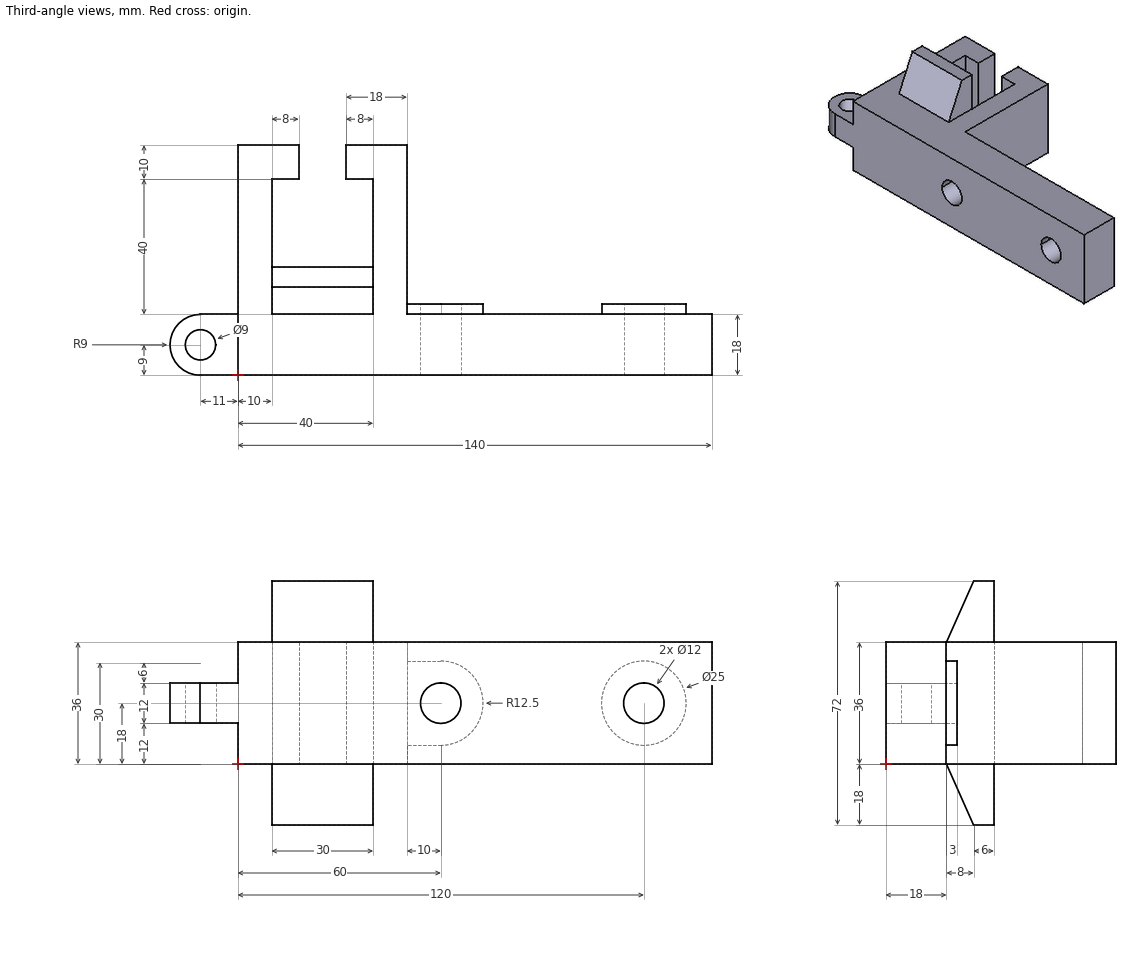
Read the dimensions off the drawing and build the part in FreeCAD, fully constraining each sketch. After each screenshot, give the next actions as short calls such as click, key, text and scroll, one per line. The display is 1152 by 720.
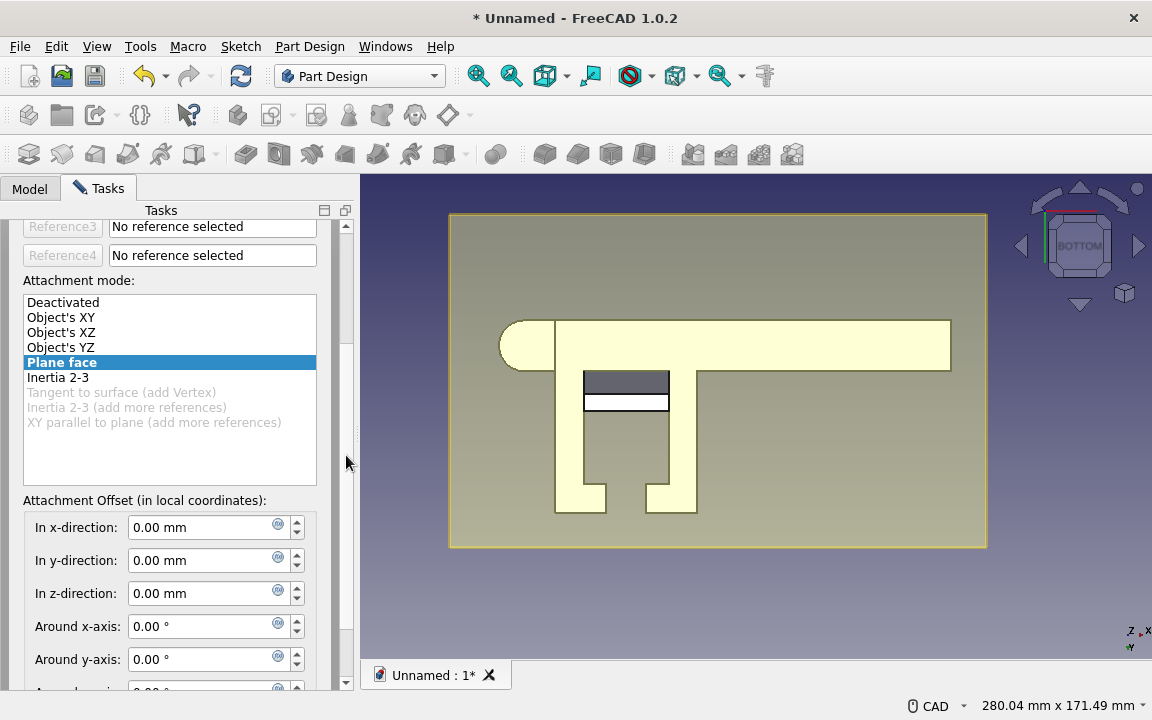
triple_click(210, 594)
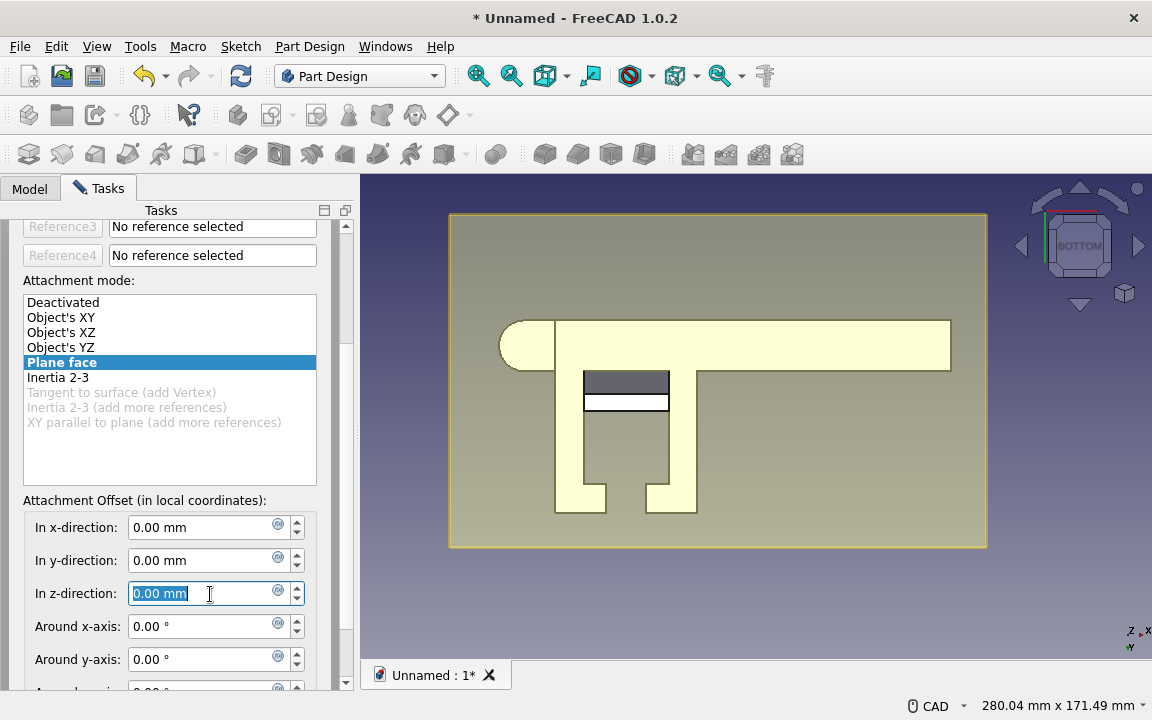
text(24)
key(Tab)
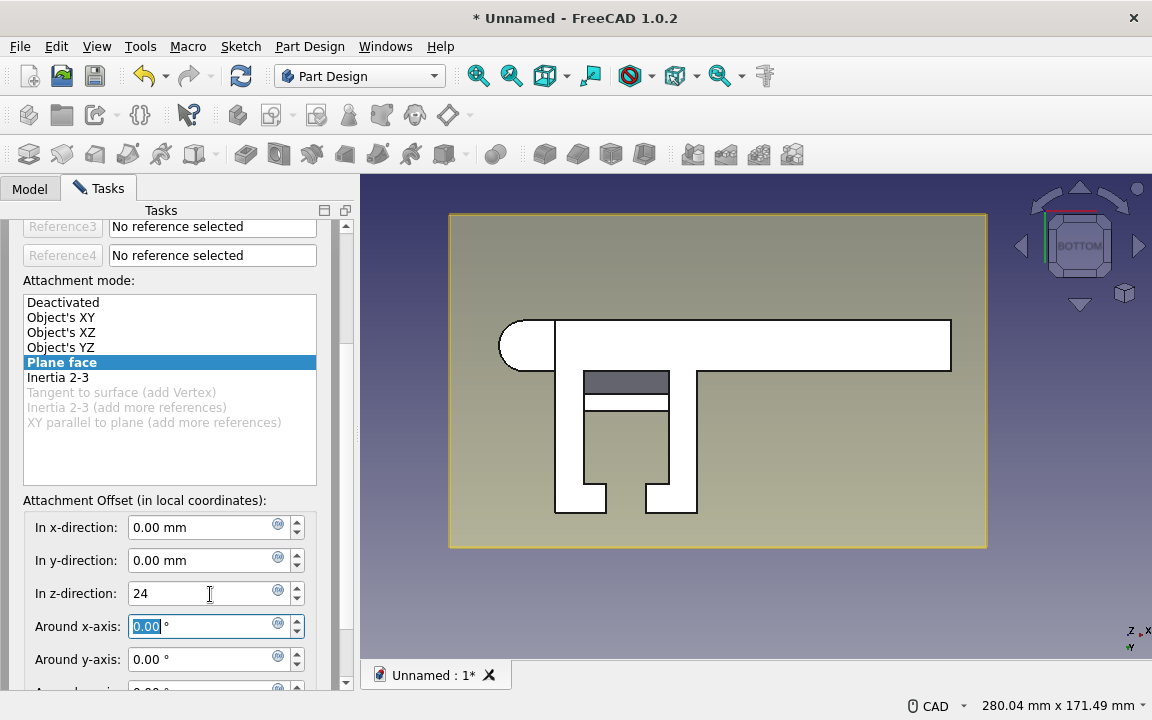
scroll(346, 455, up, 4)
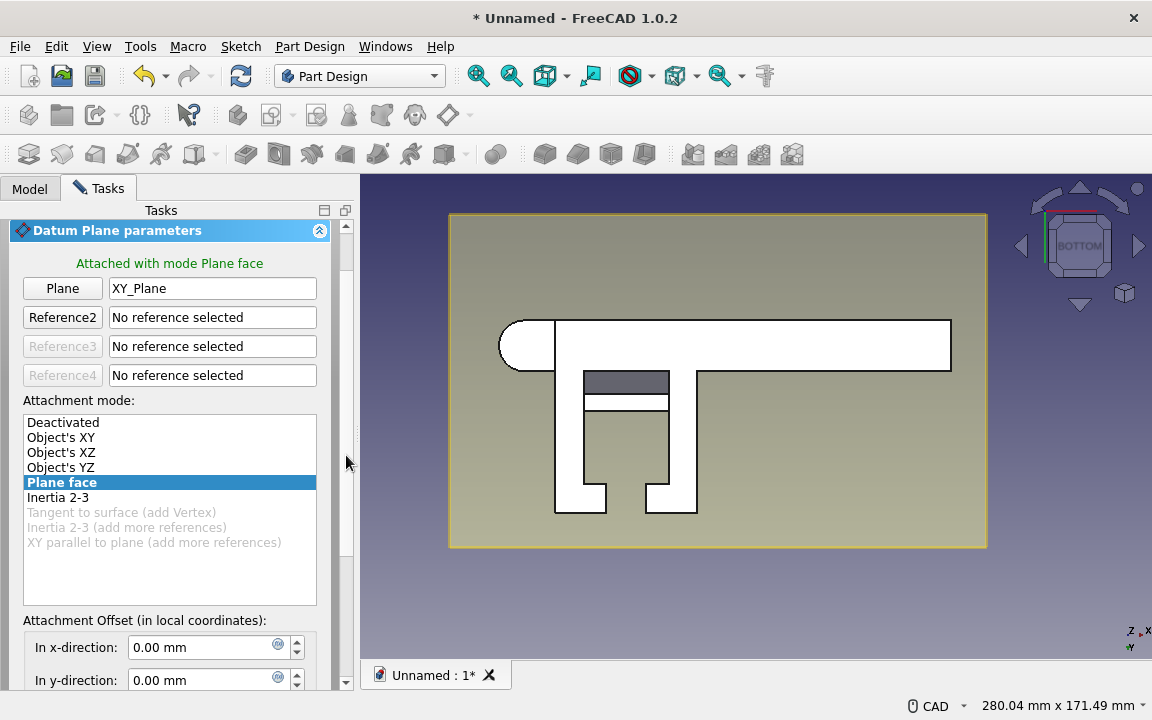
click(127, 249)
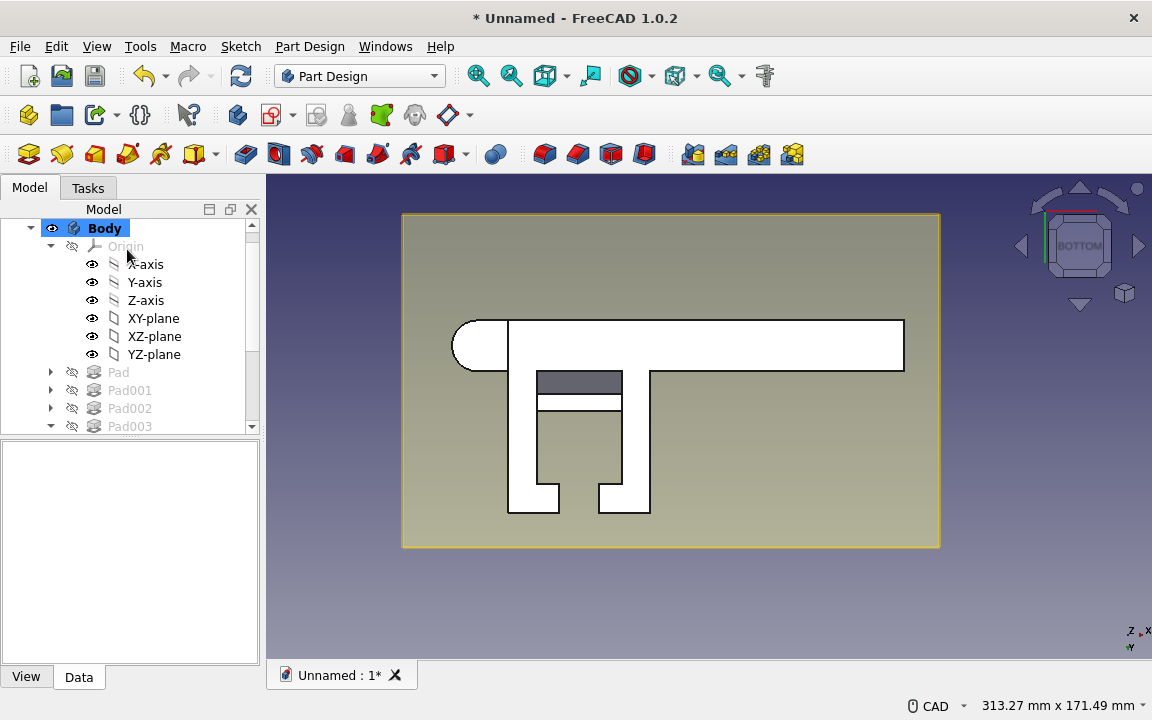
scroll(121, 332, down, 3)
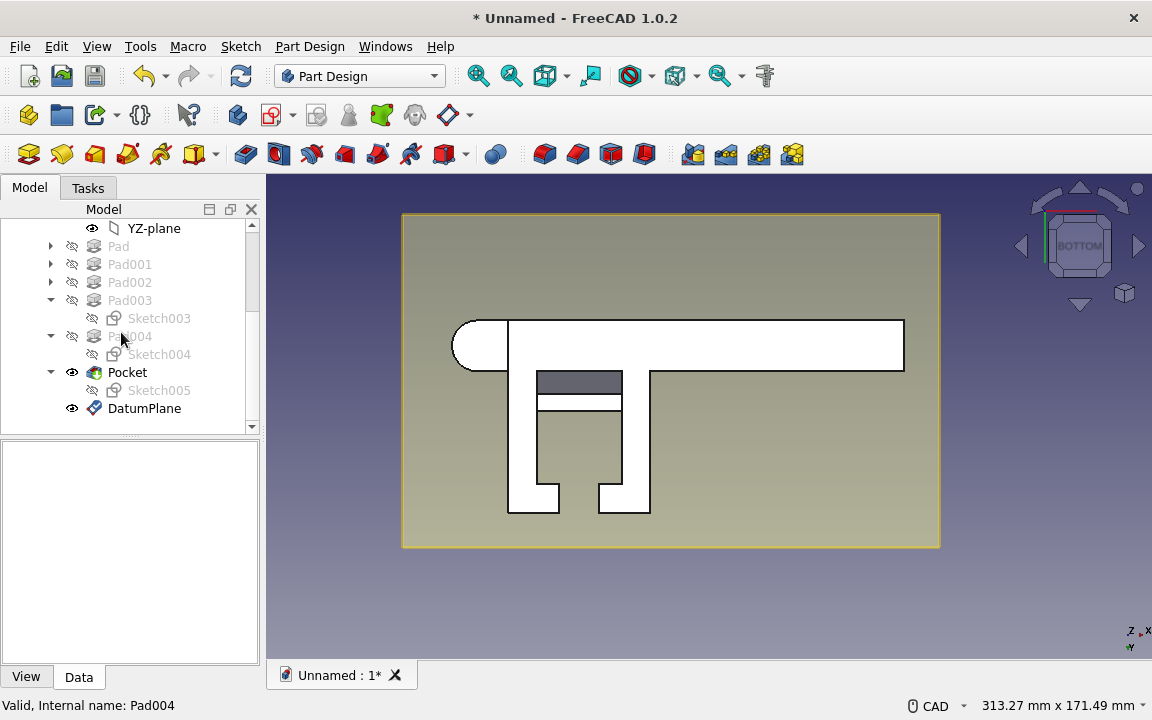
click(117, 408)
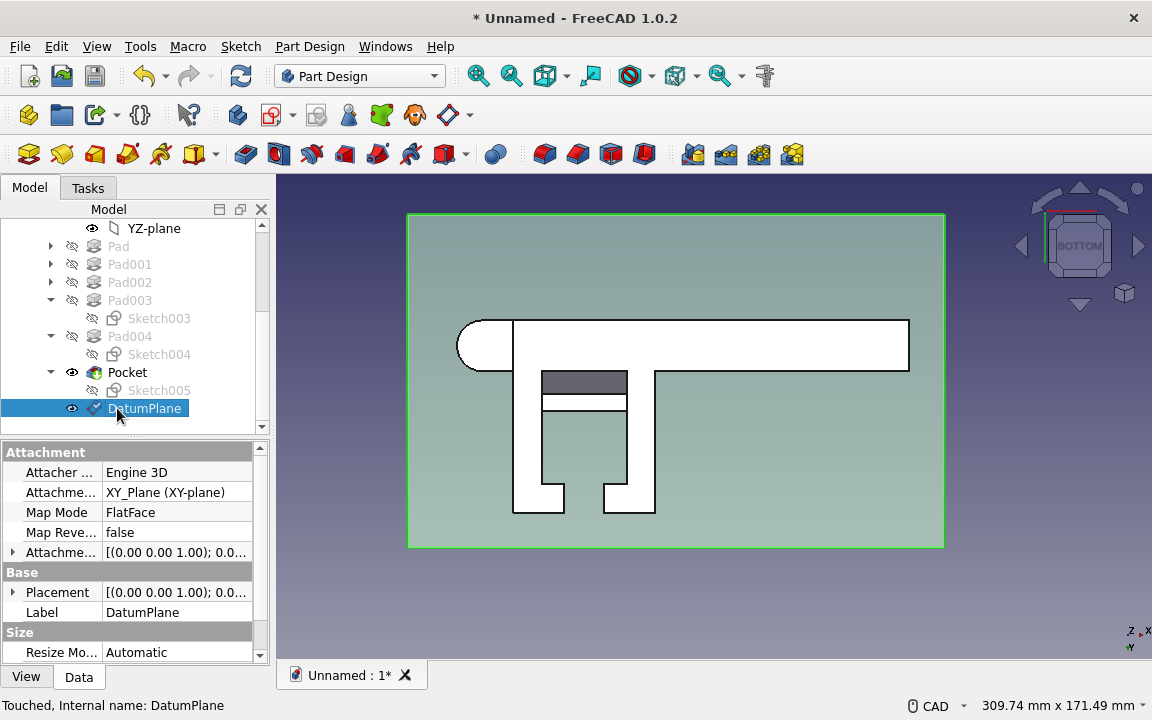
click(270, 116)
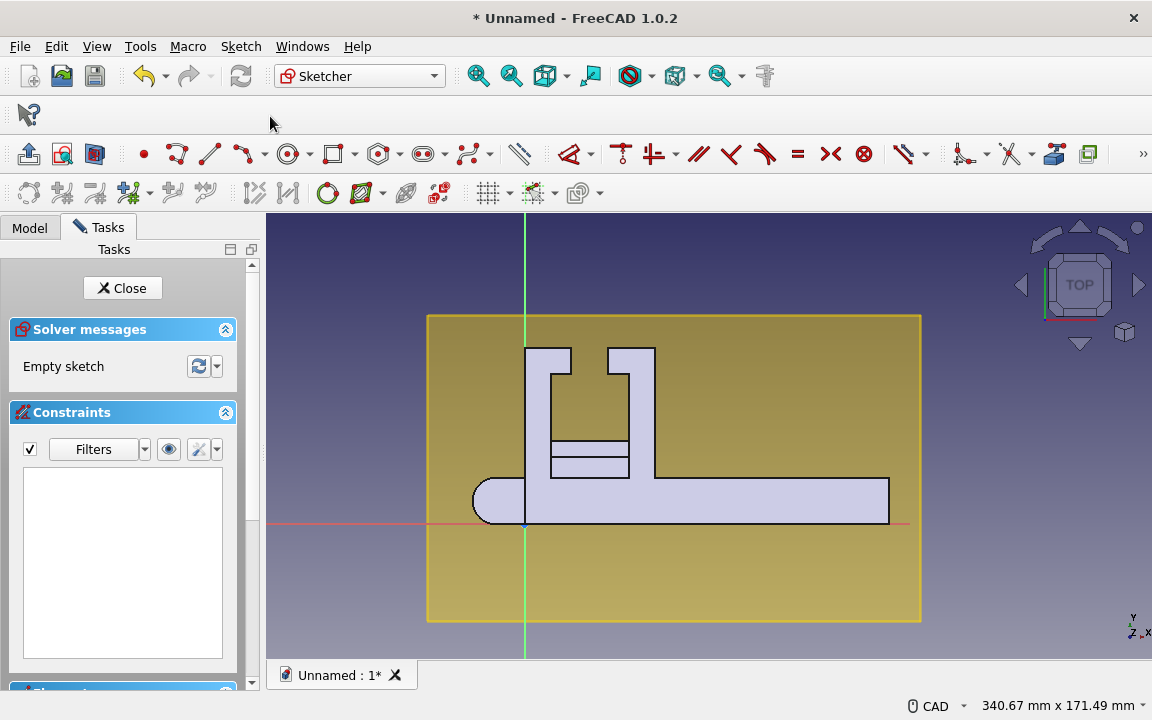
key(q)
key(s)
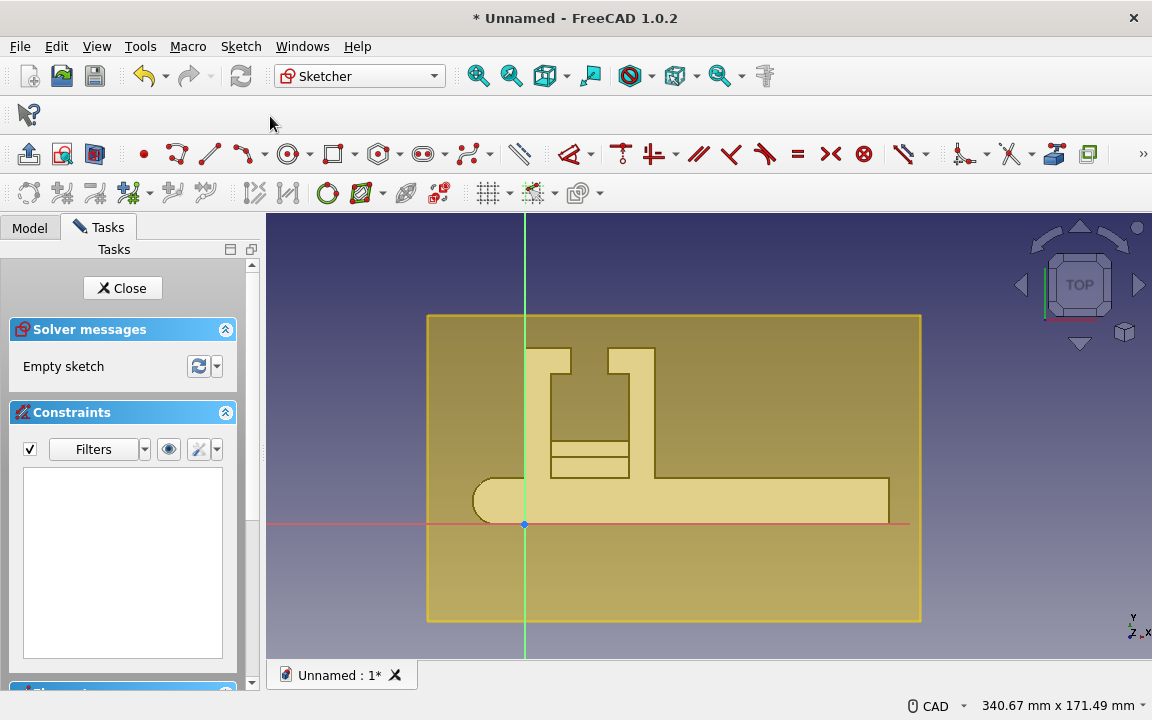
scroll(471, 514, up, 9)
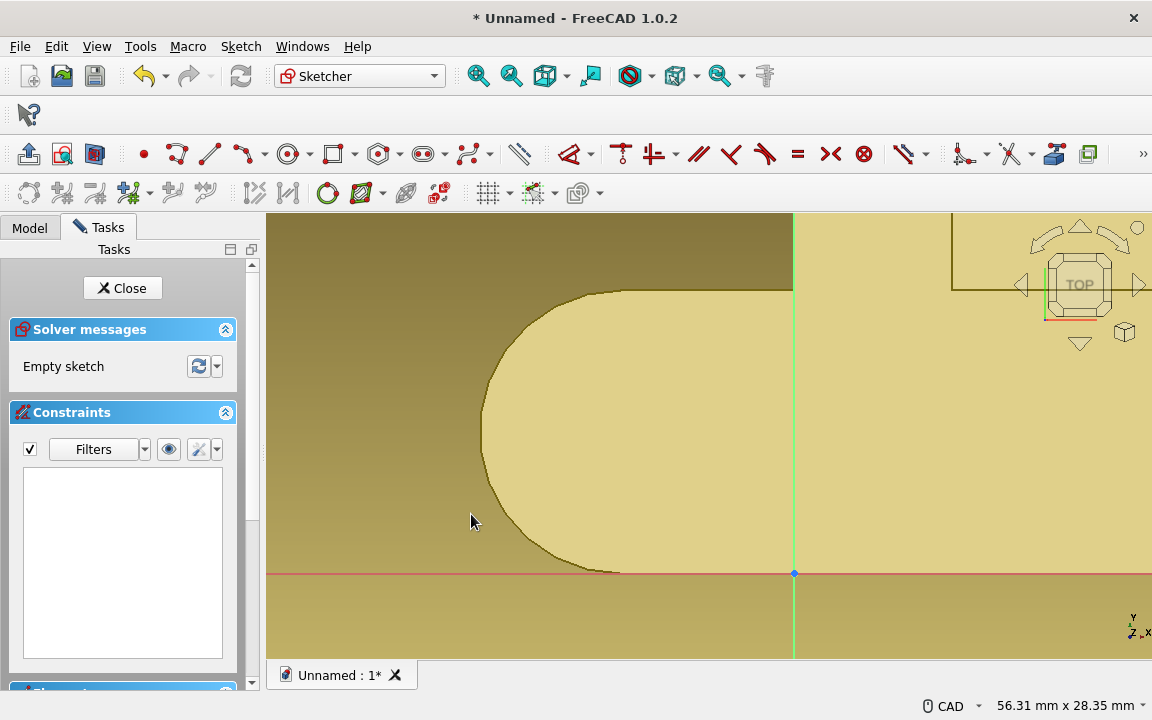
click(177, 154)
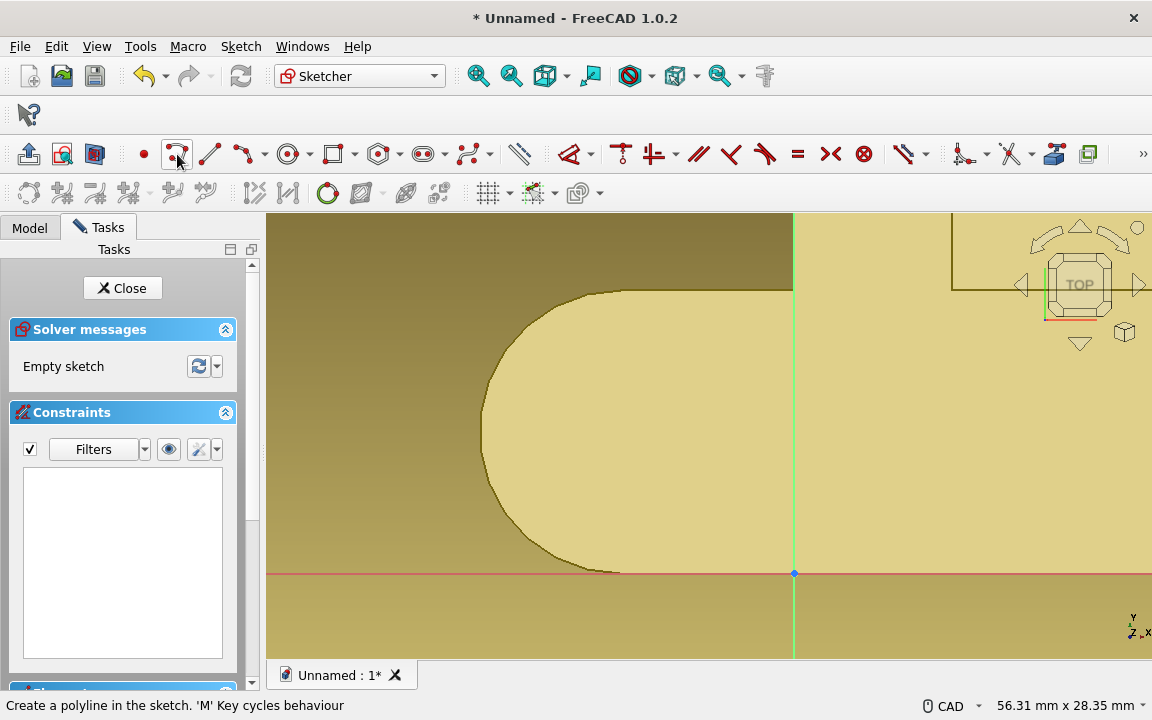
click(621, 574)
click(794, 574)
click(785, 290)
click(621, 290)
right_click(621, 290)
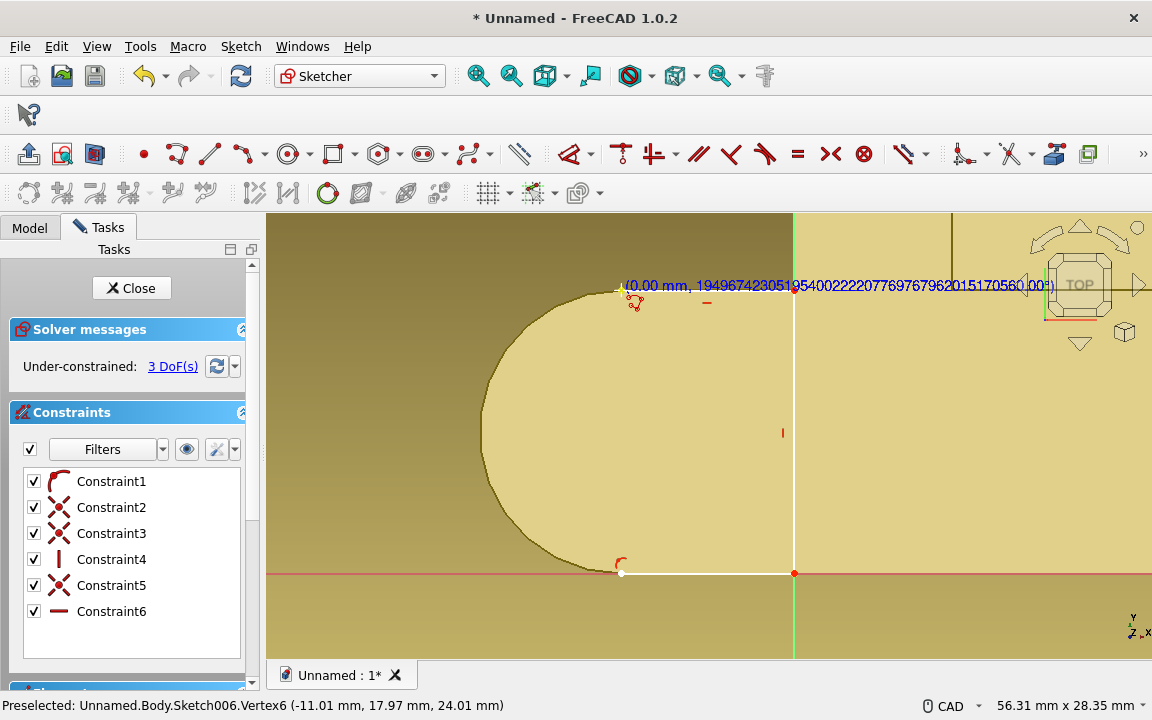
key(g)
key(3)
key(a)